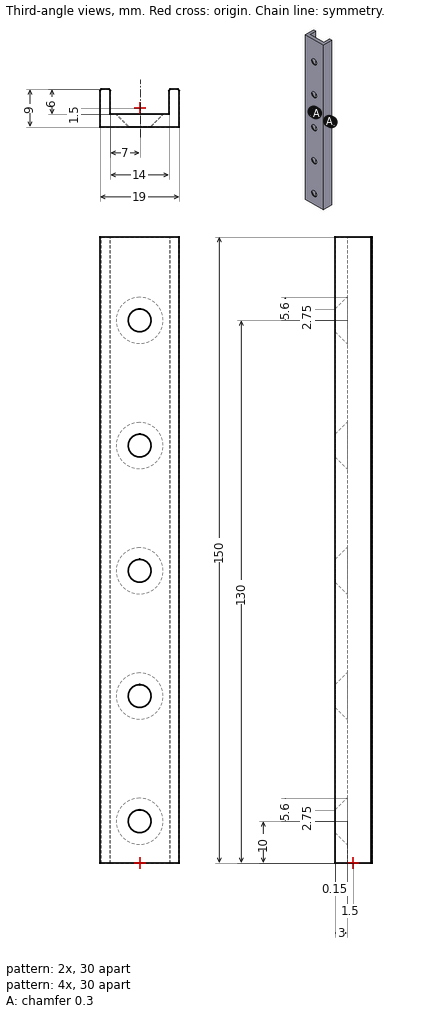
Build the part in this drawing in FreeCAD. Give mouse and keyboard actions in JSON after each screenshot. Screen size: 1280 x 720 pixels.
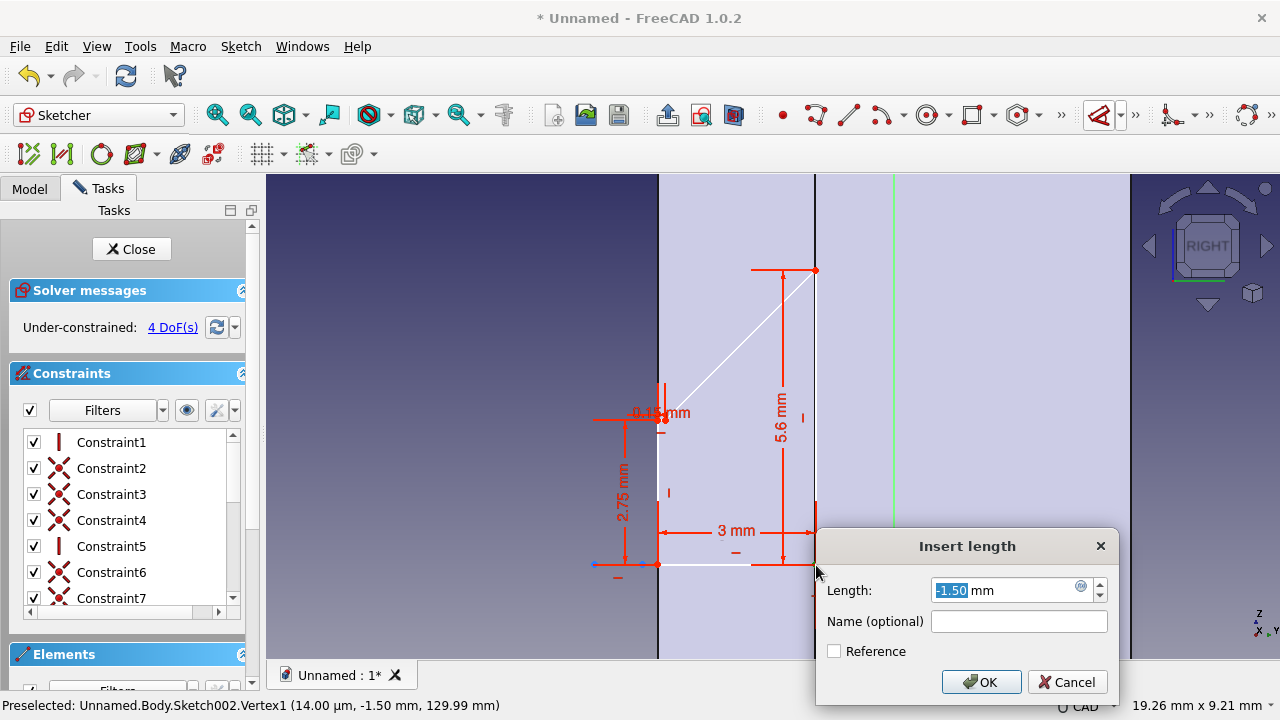
{"action": "type", "text": "-1.5"}
{"action": "key", "text": "Return"}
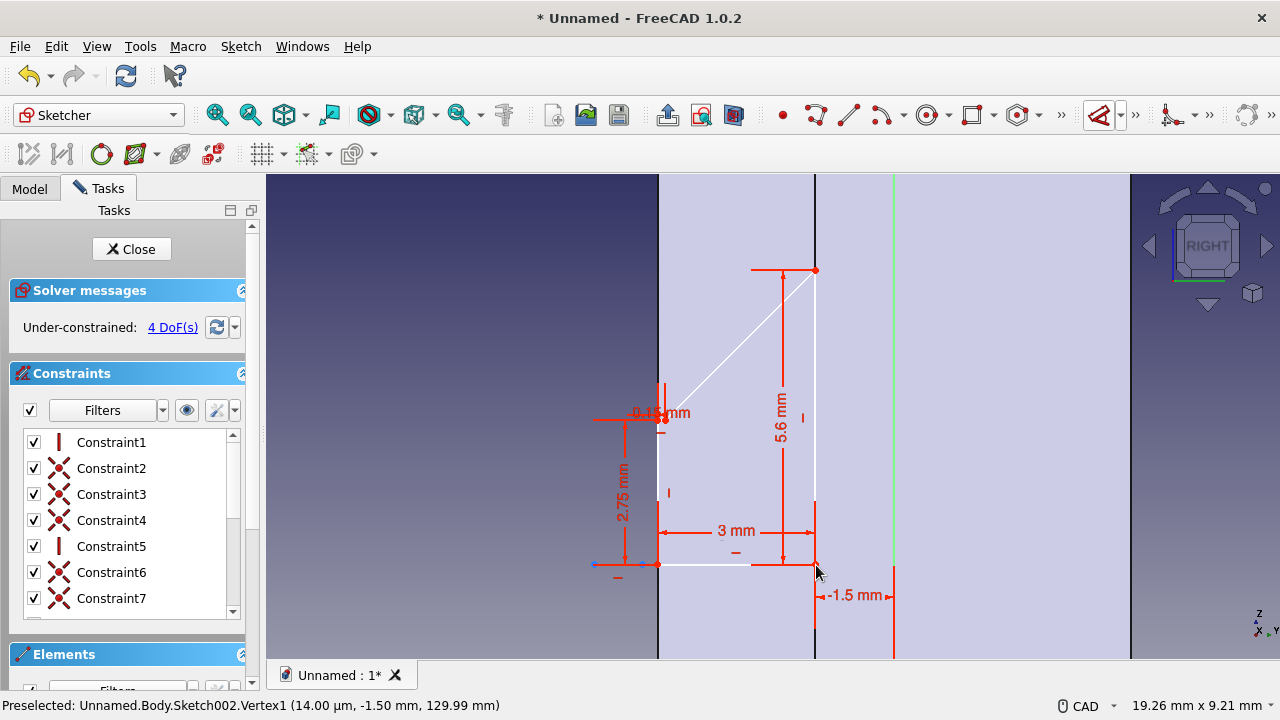
{"action": "left_click", "coordinate": [815, 565]}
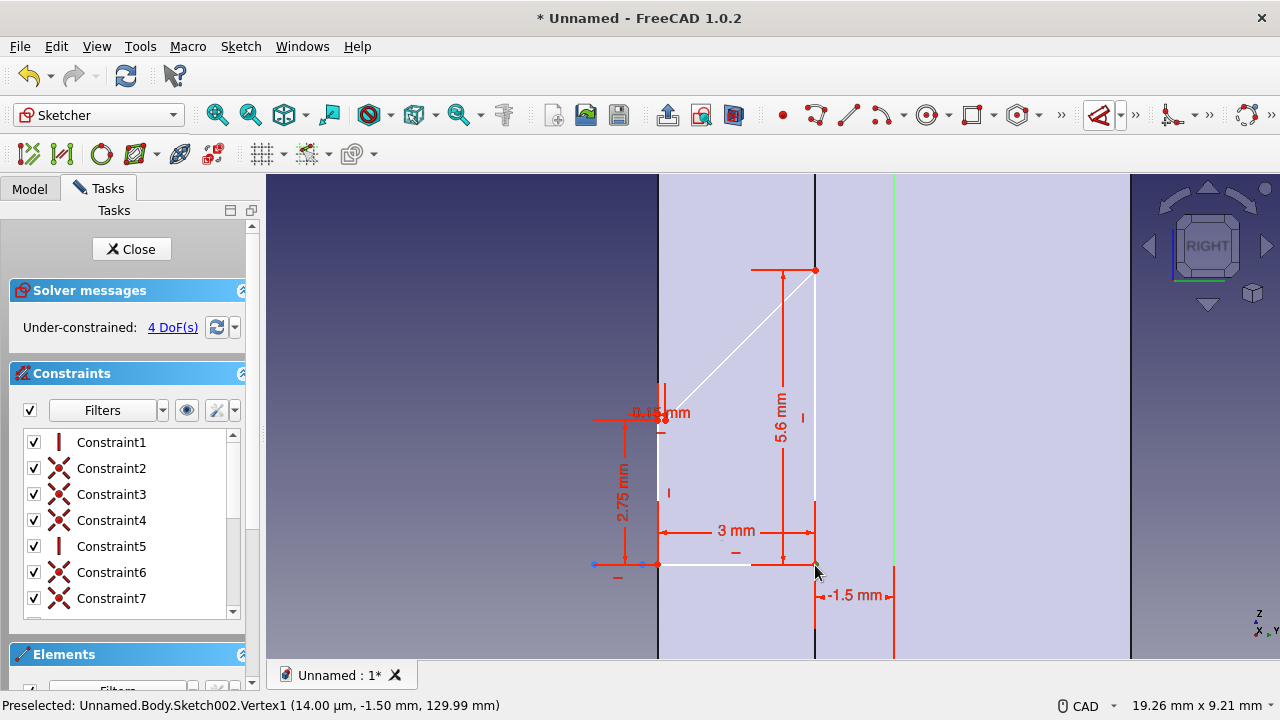
{"action": "left_click", "coordinate": [1120, 116]}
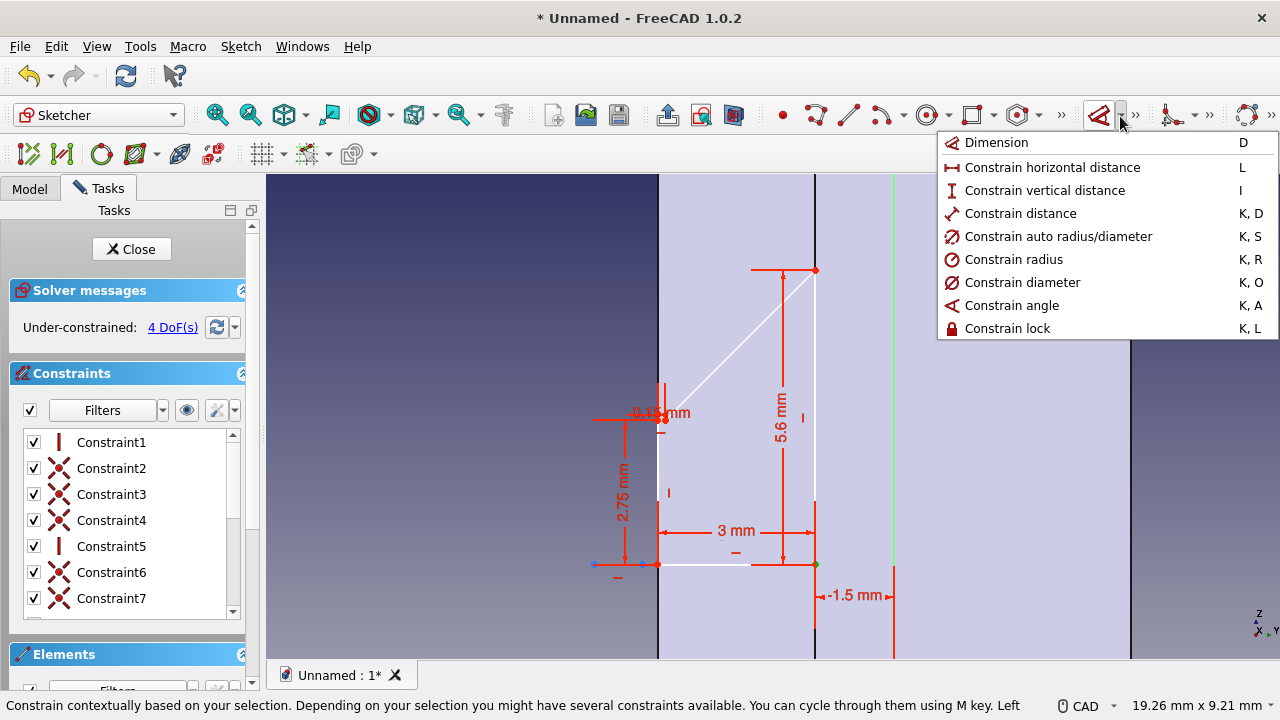
{"action": "left_click", "coordinate": [1108, 190]}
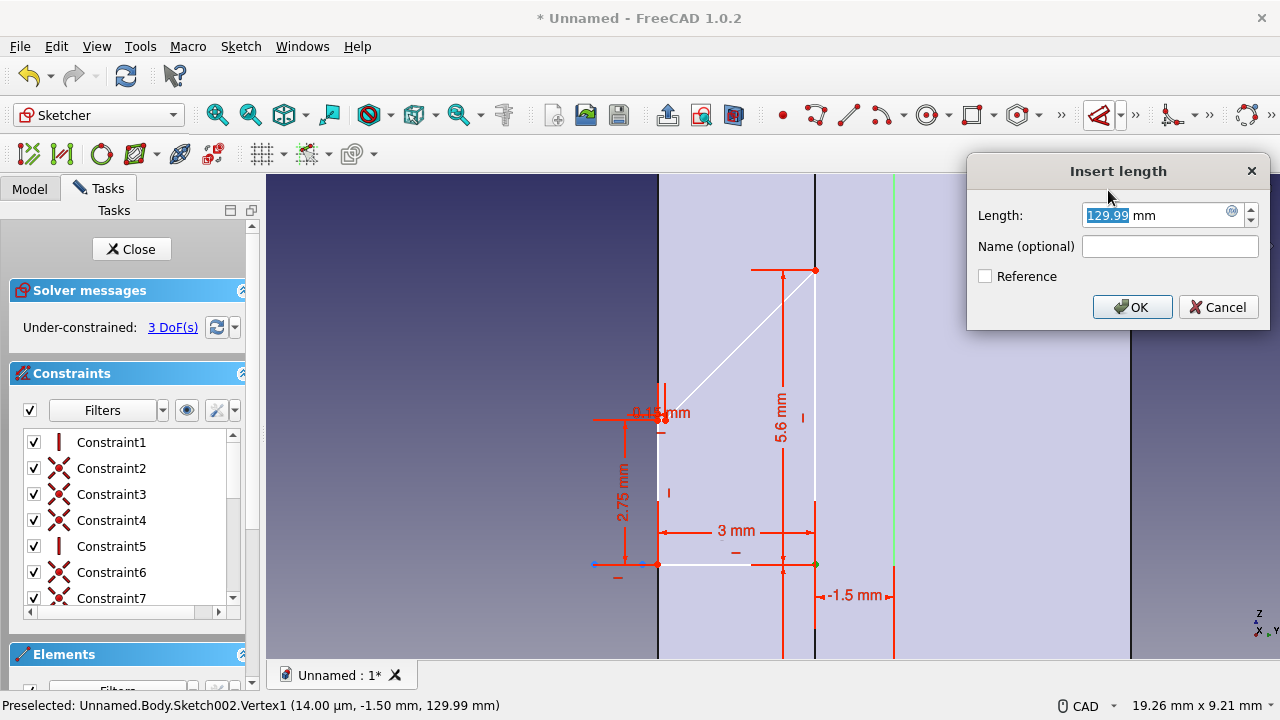
{"action": "type", "text": "130"}
{"action": "key", "text": "Return"}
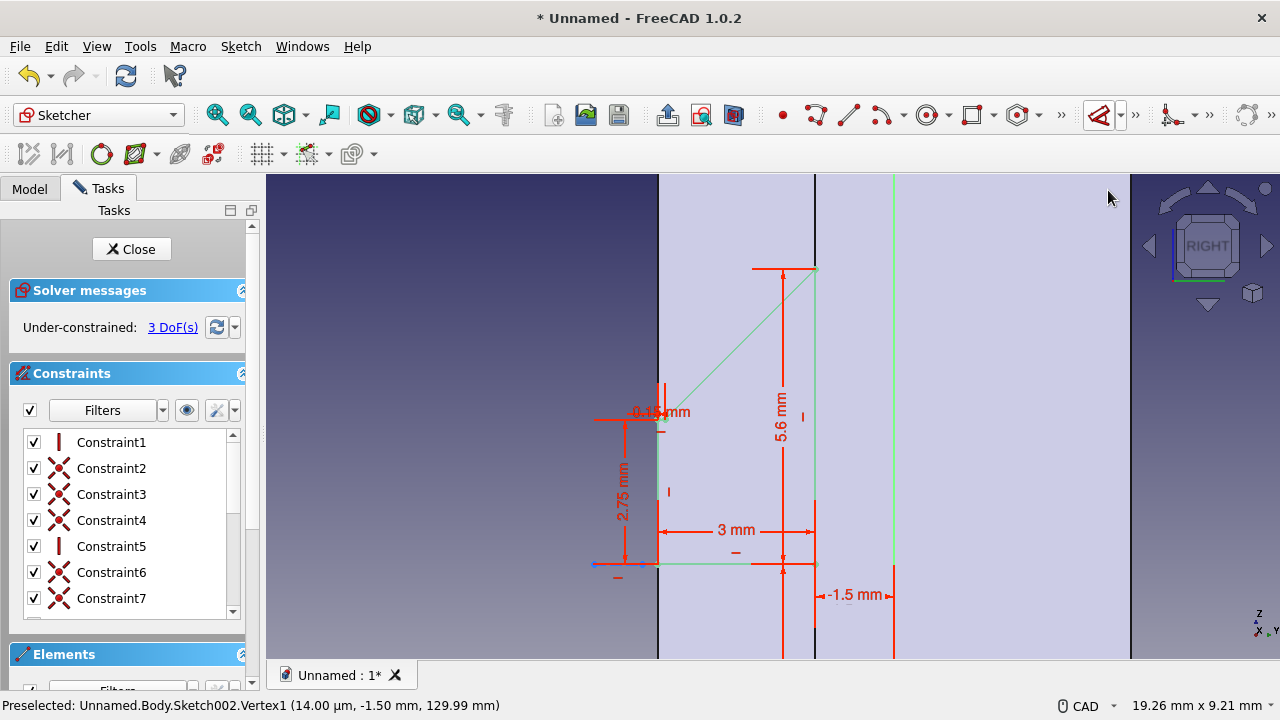
{"action": "left_click", "coordinate": [642, 565]}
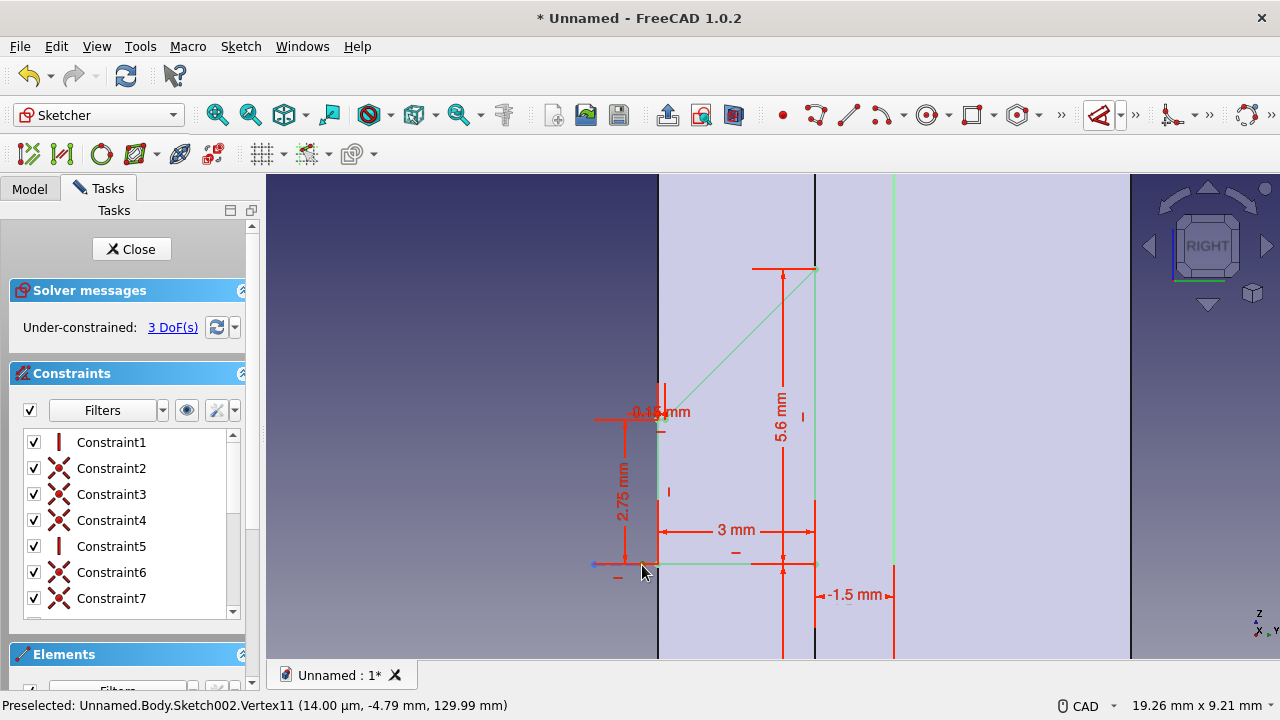
{"action": "left_click", "coordinate": [1120, 116]}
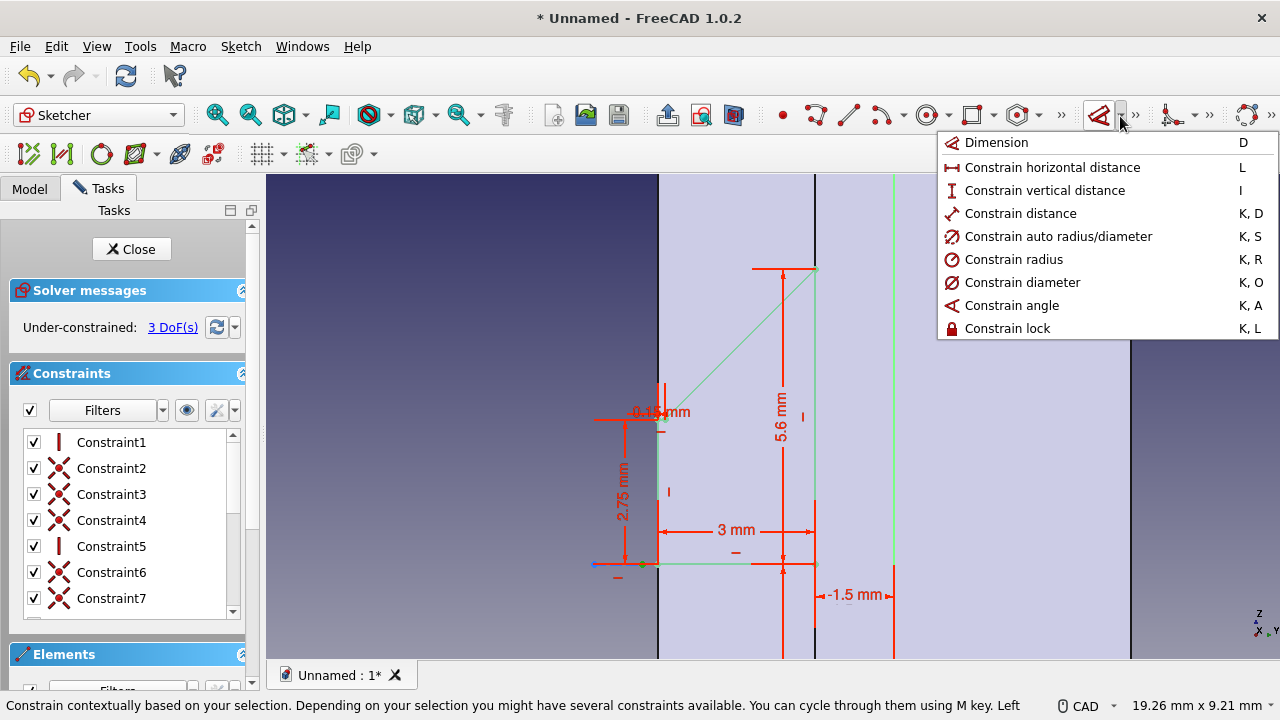
{"action": "left_click", "coordinate": [1108, 190]}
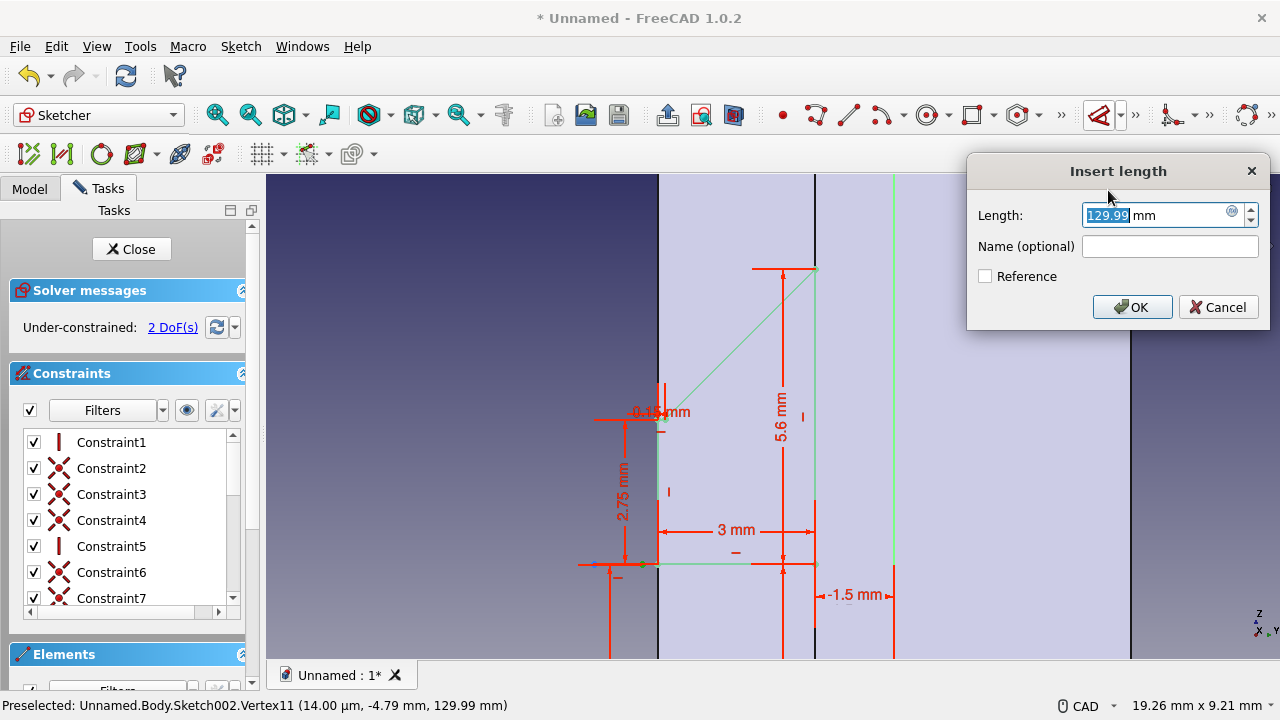
{"action": "type", "text": "130"}
{"action": "key", "text": "Return"}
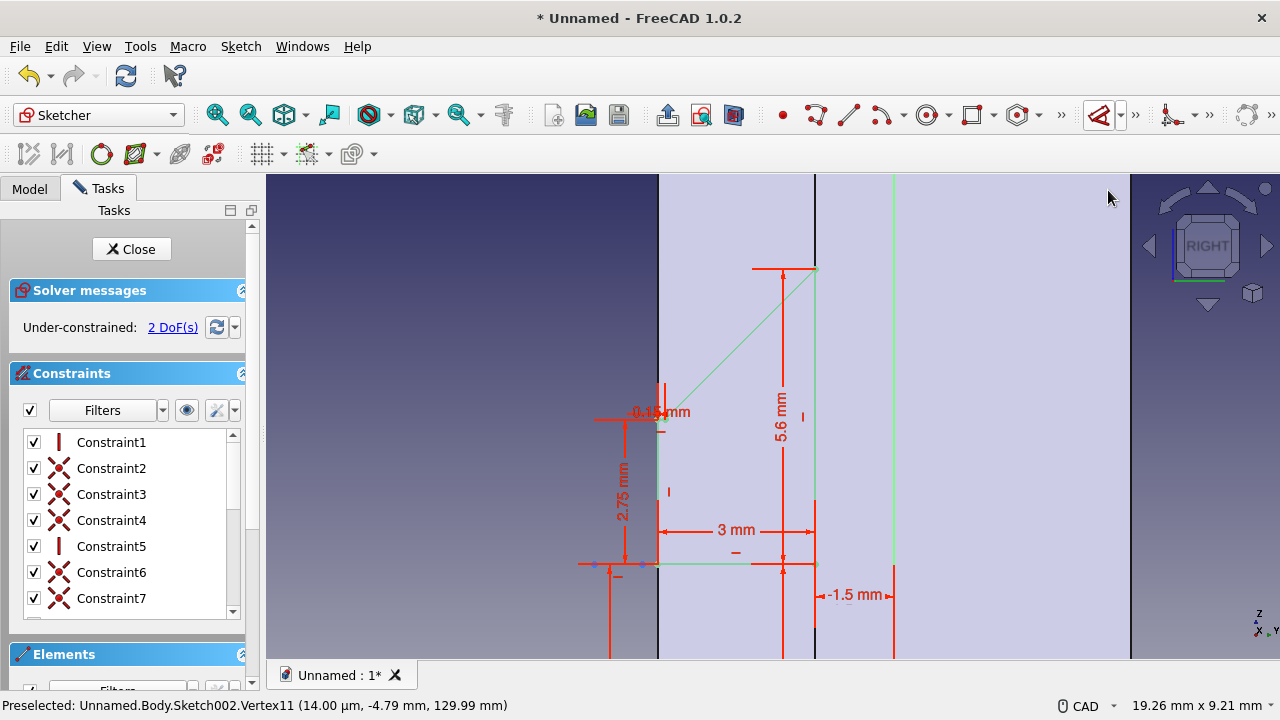
{"action": "left_click", "coordinate": [132, 249]}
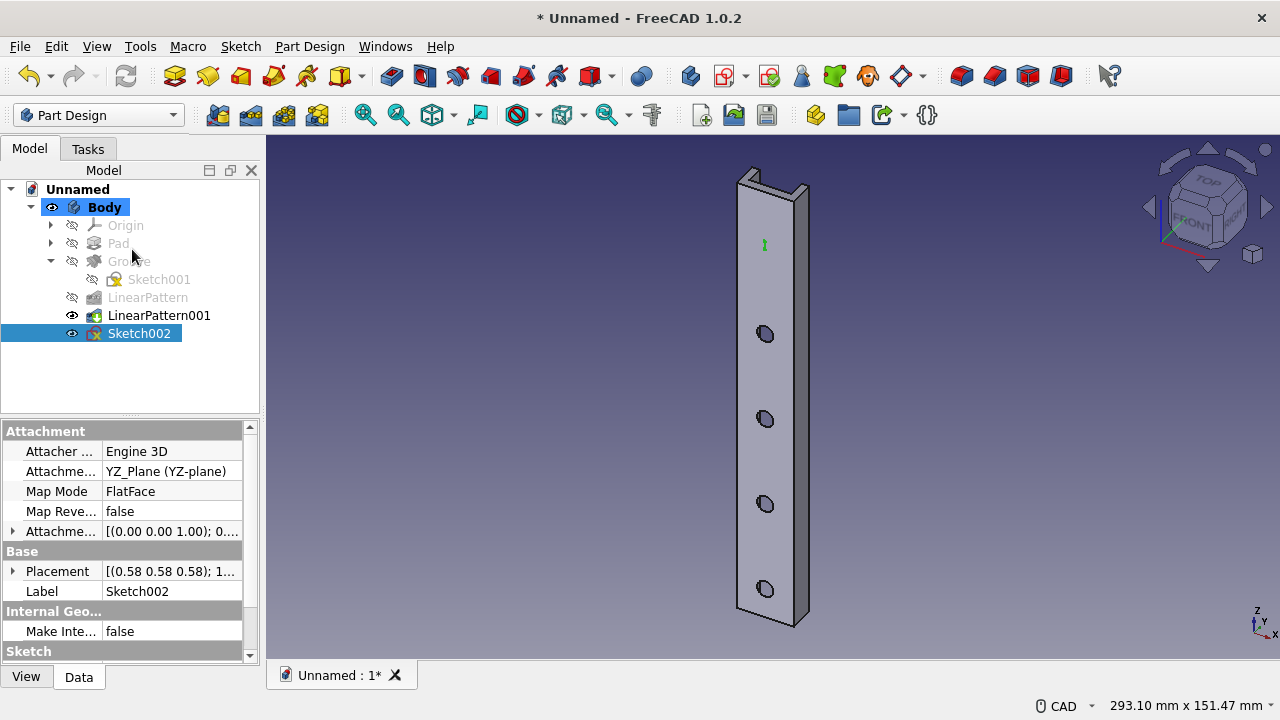
{"action": "left_click", "coordinate": [458, 76]}